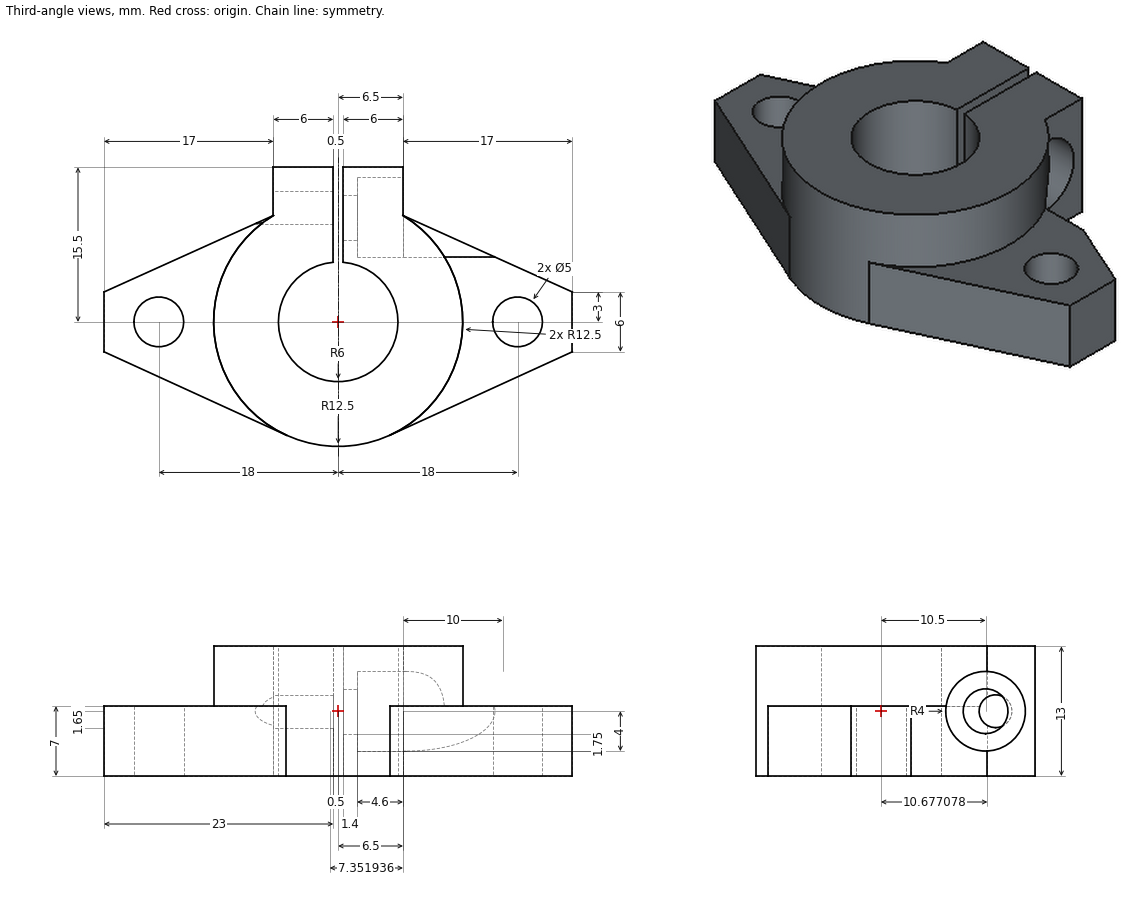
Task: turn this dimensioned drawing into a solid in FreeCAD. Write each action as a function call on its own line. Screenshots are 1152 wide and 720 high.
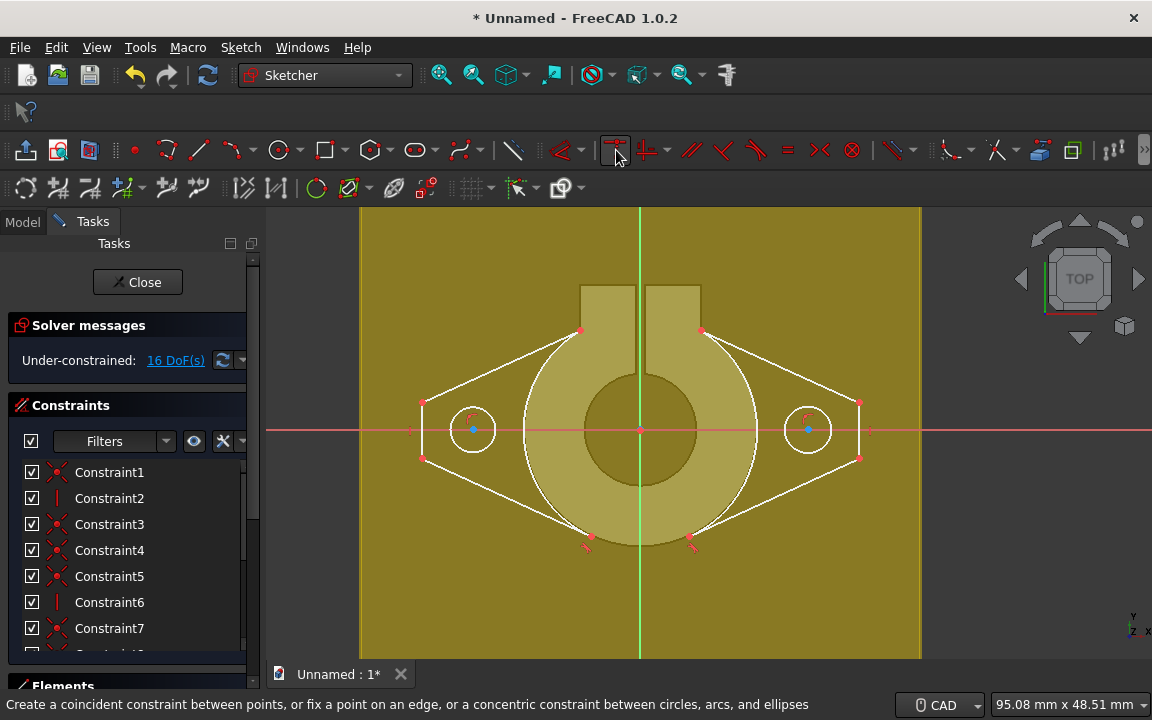
scroll(640, 430, up, 3)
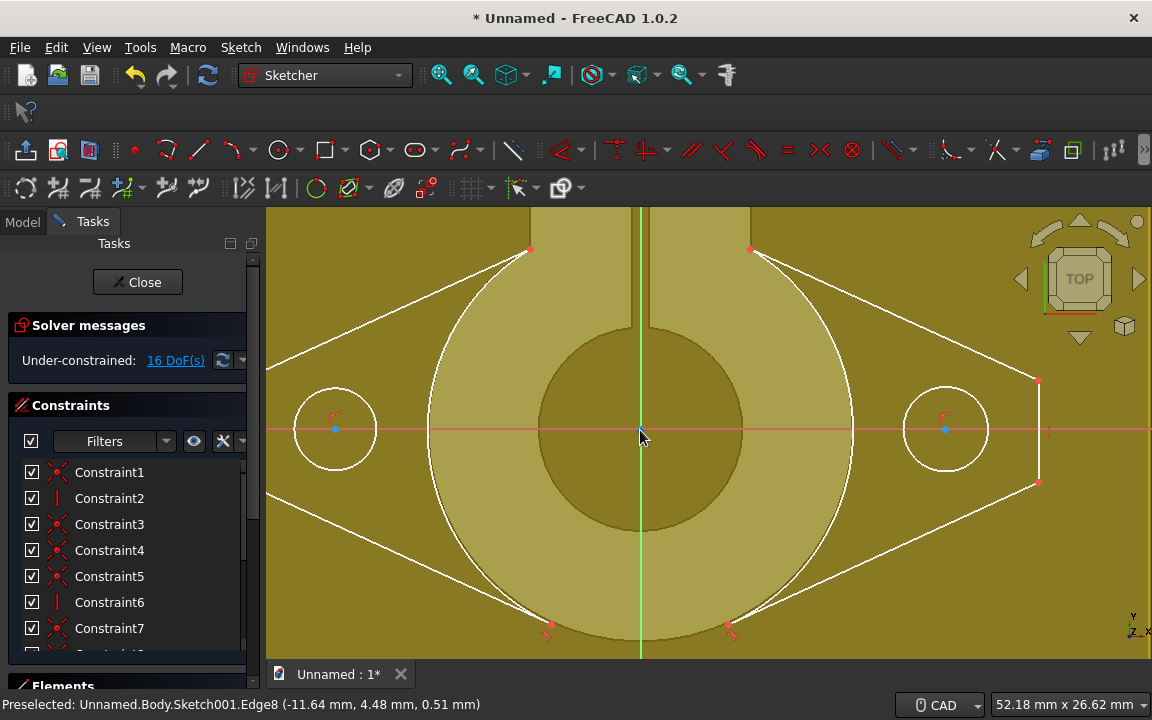
drag(630, 419, 651, 441)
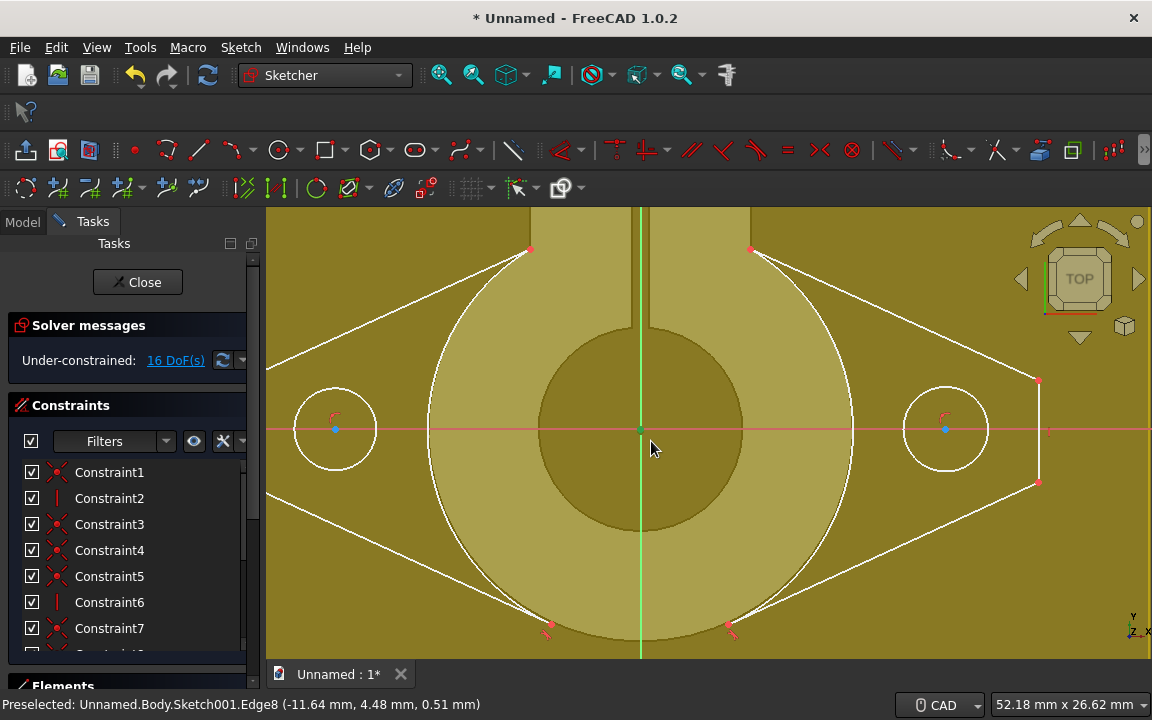
click(616, 150)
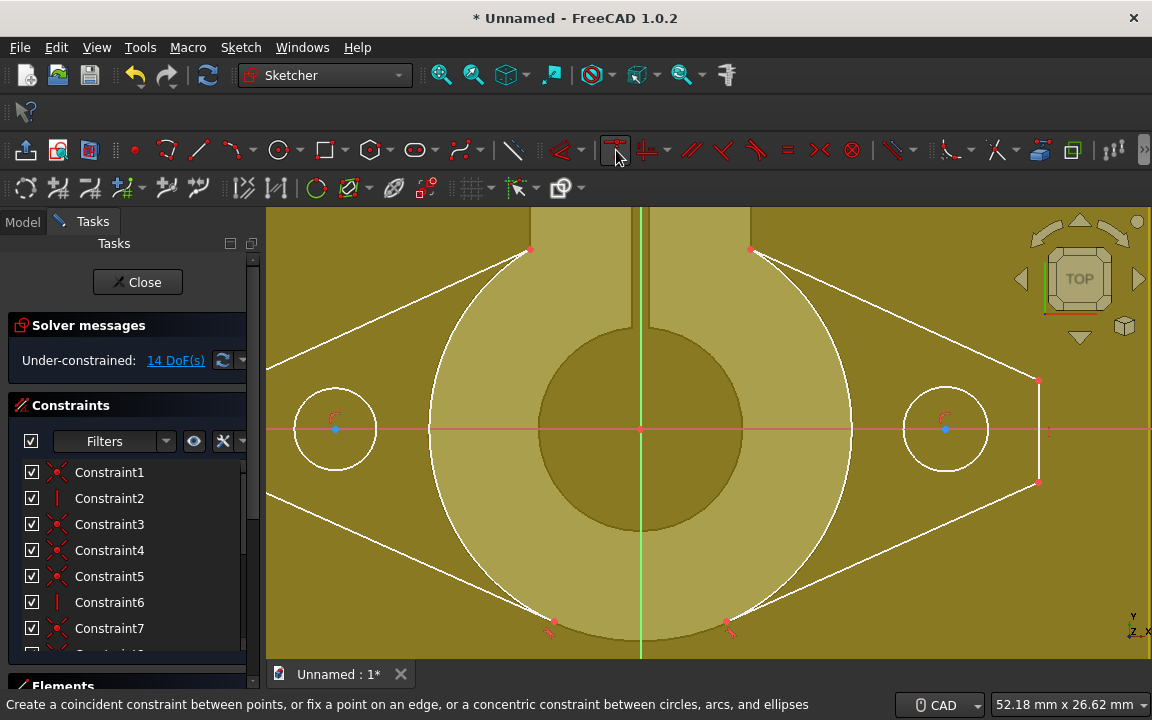
click(826, 530)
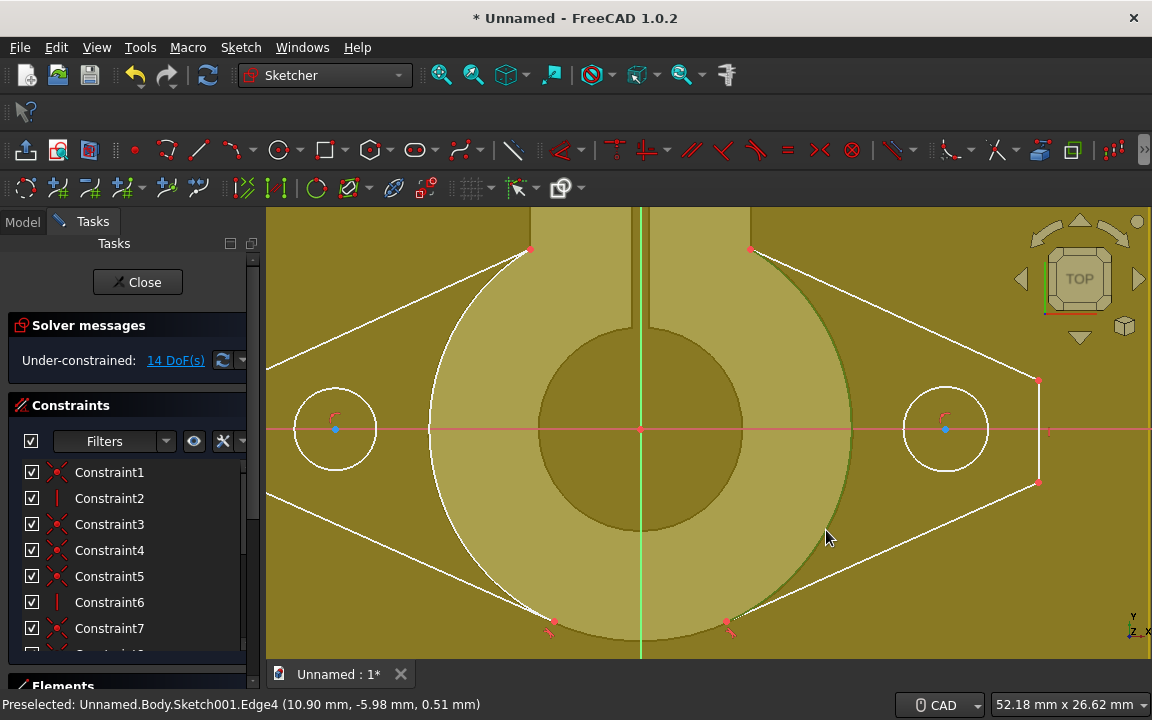
click(444, 353)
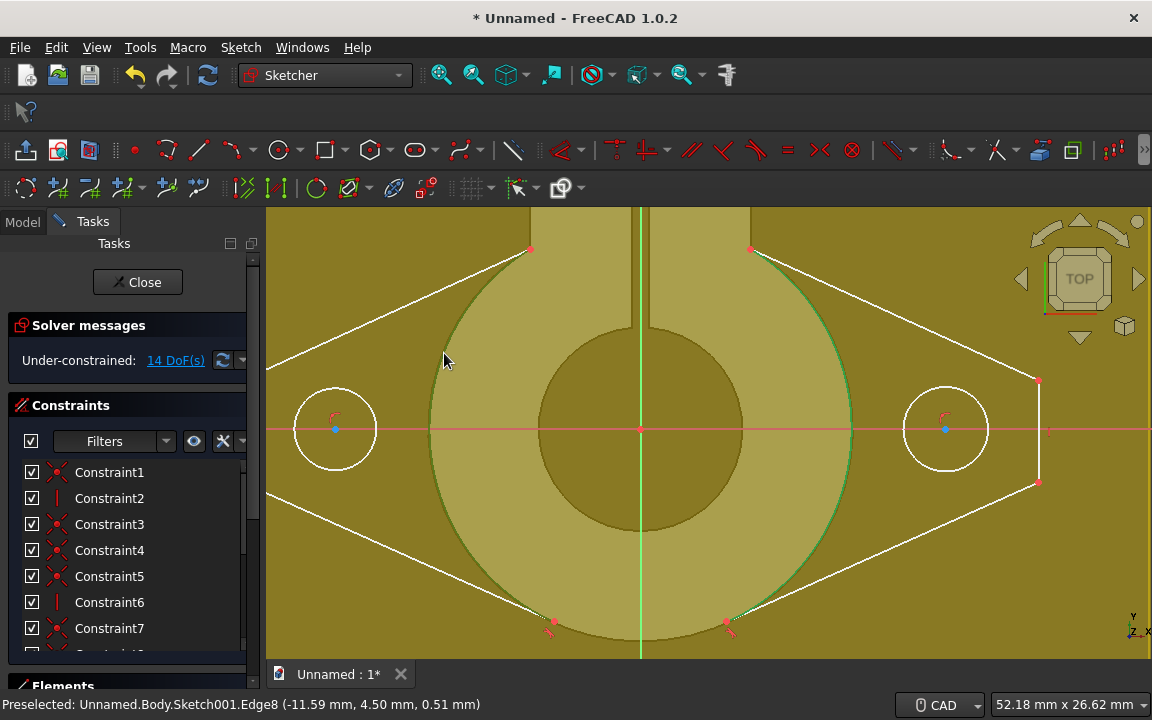
click(788, 150)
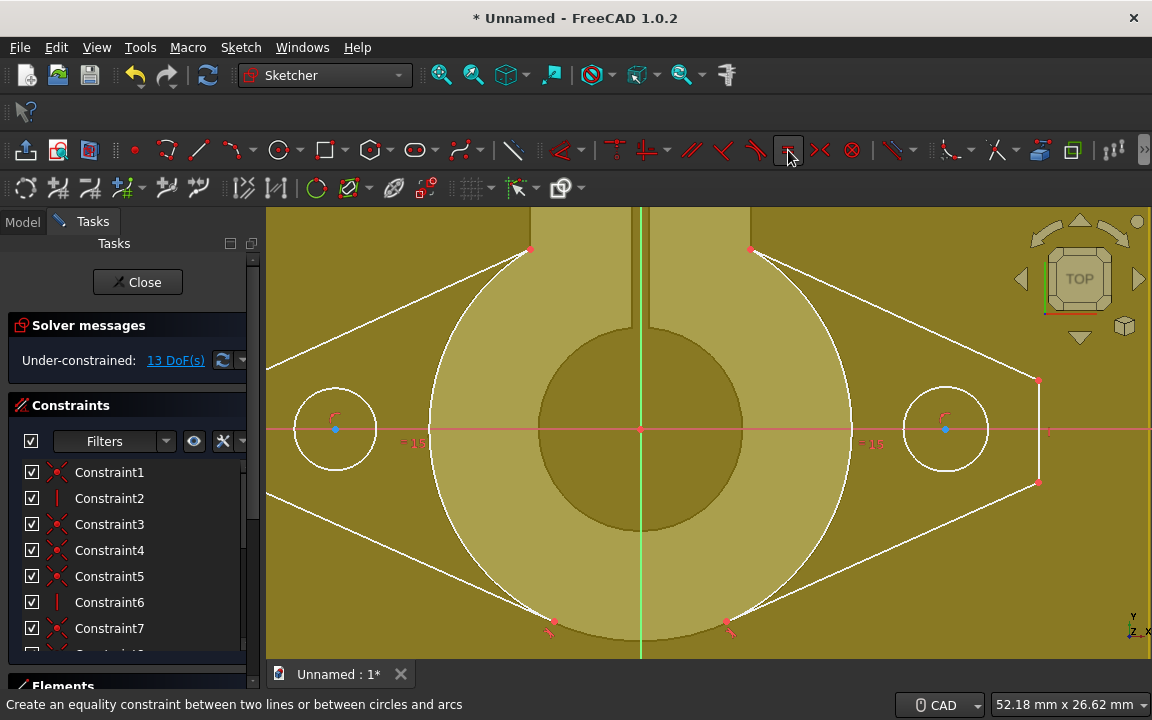
click(976, 399)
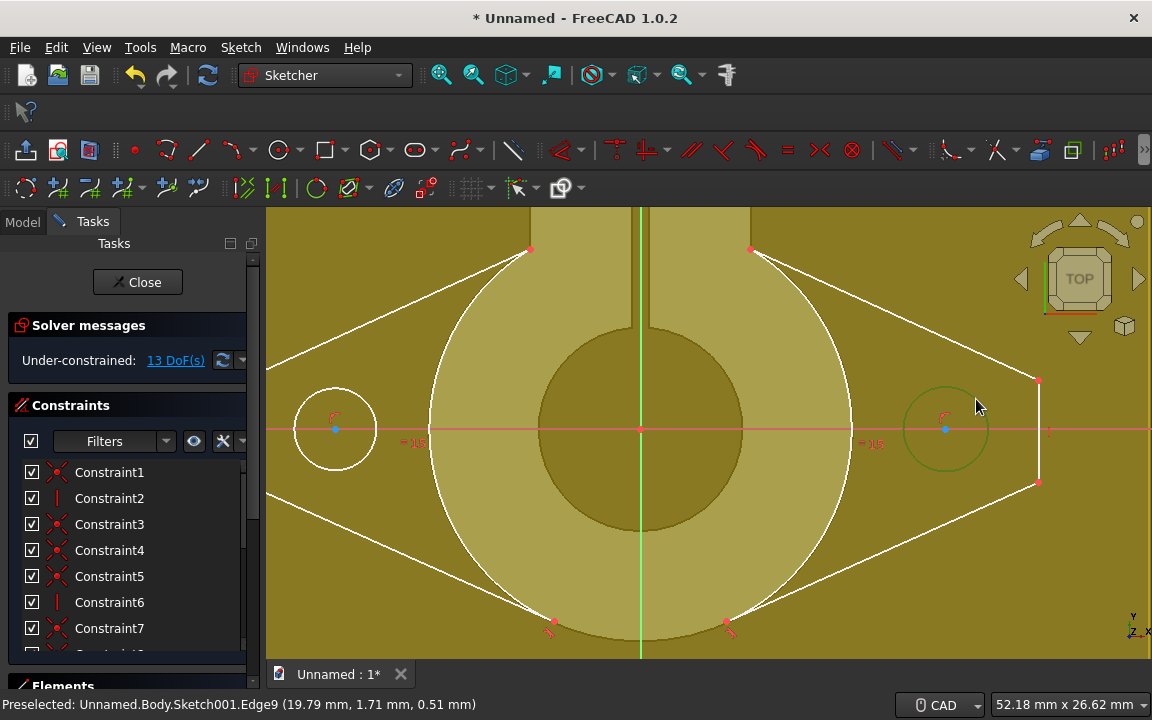
click(364, 400)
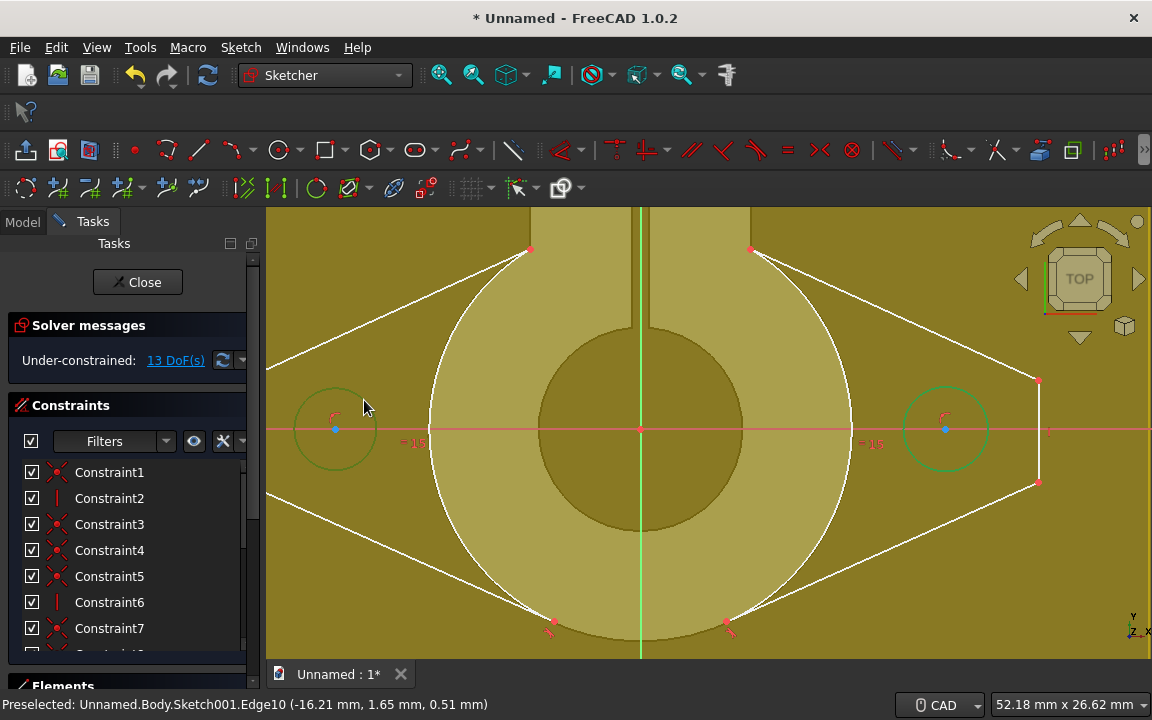
click(788, 150)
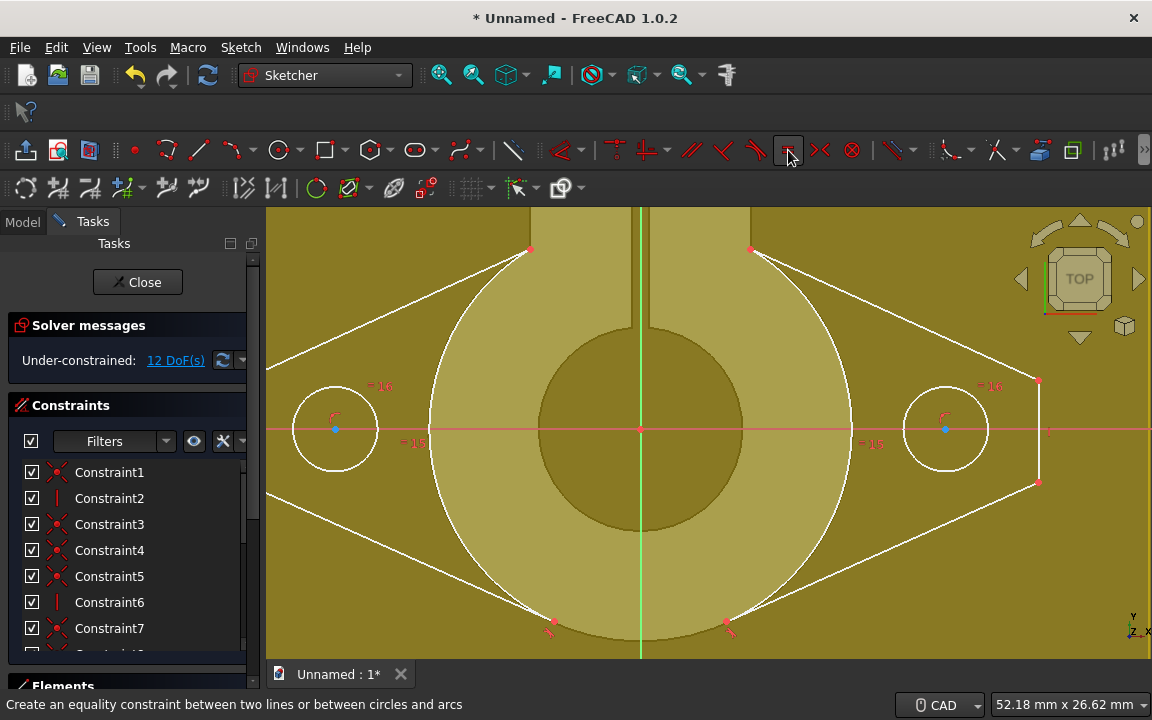
scroll(640, 429, down, 2)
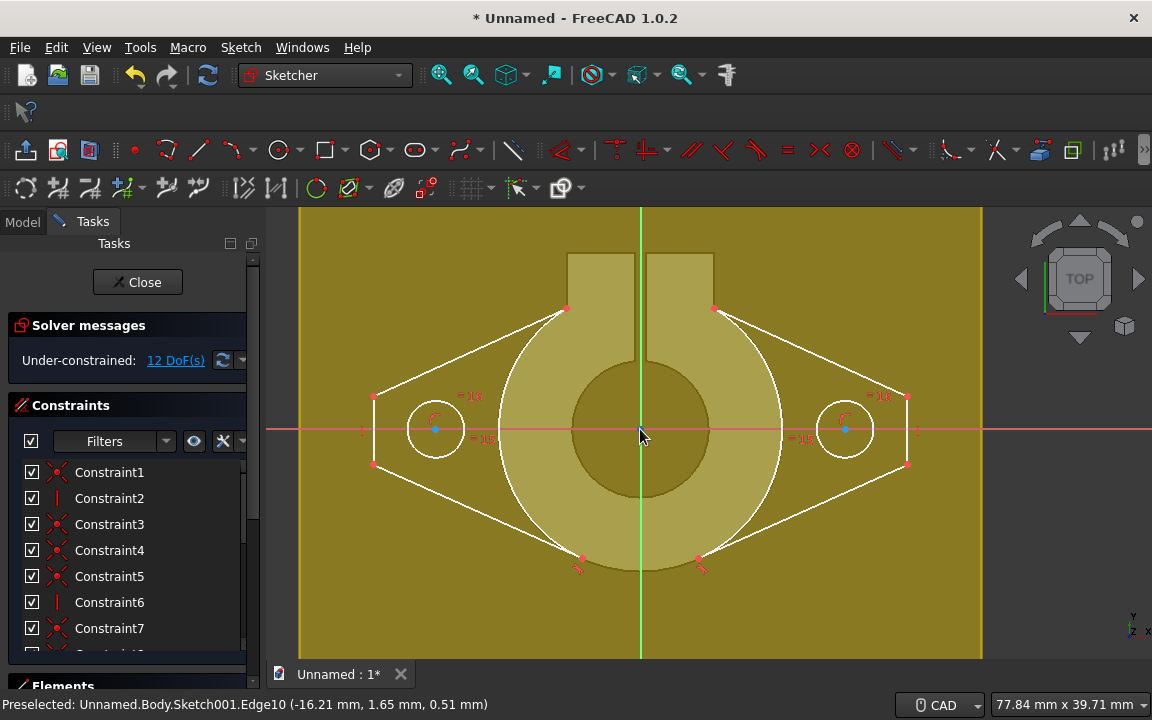
click(907, 465)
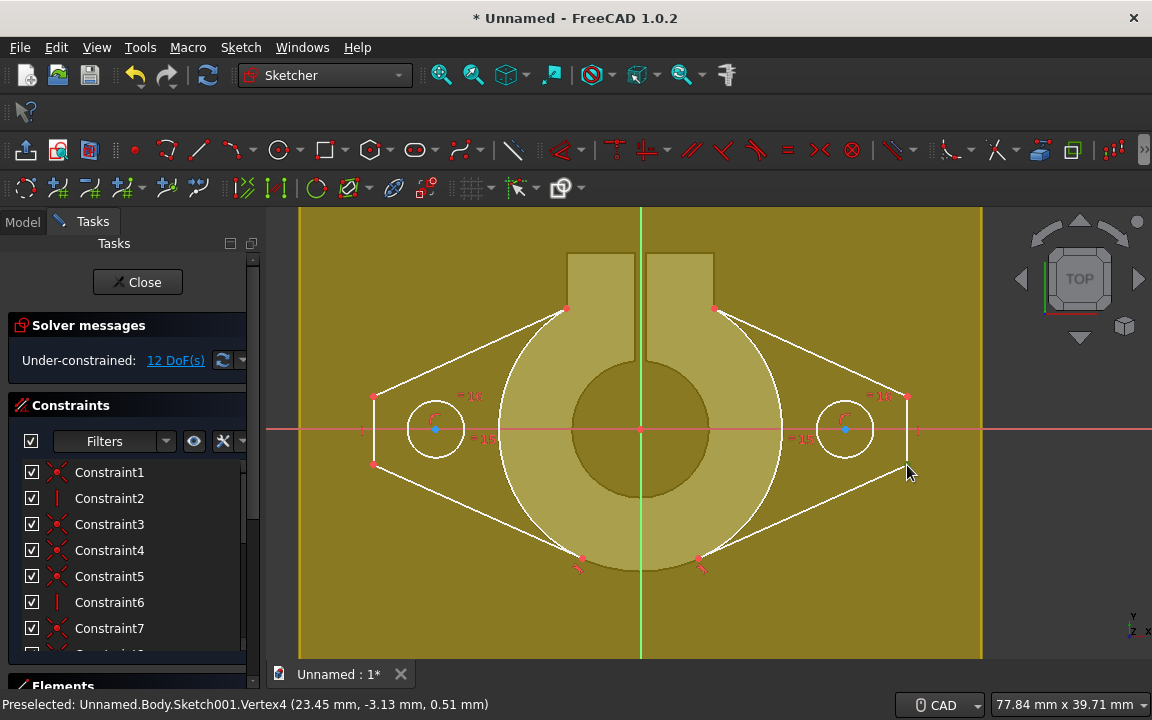
click(374, 465)